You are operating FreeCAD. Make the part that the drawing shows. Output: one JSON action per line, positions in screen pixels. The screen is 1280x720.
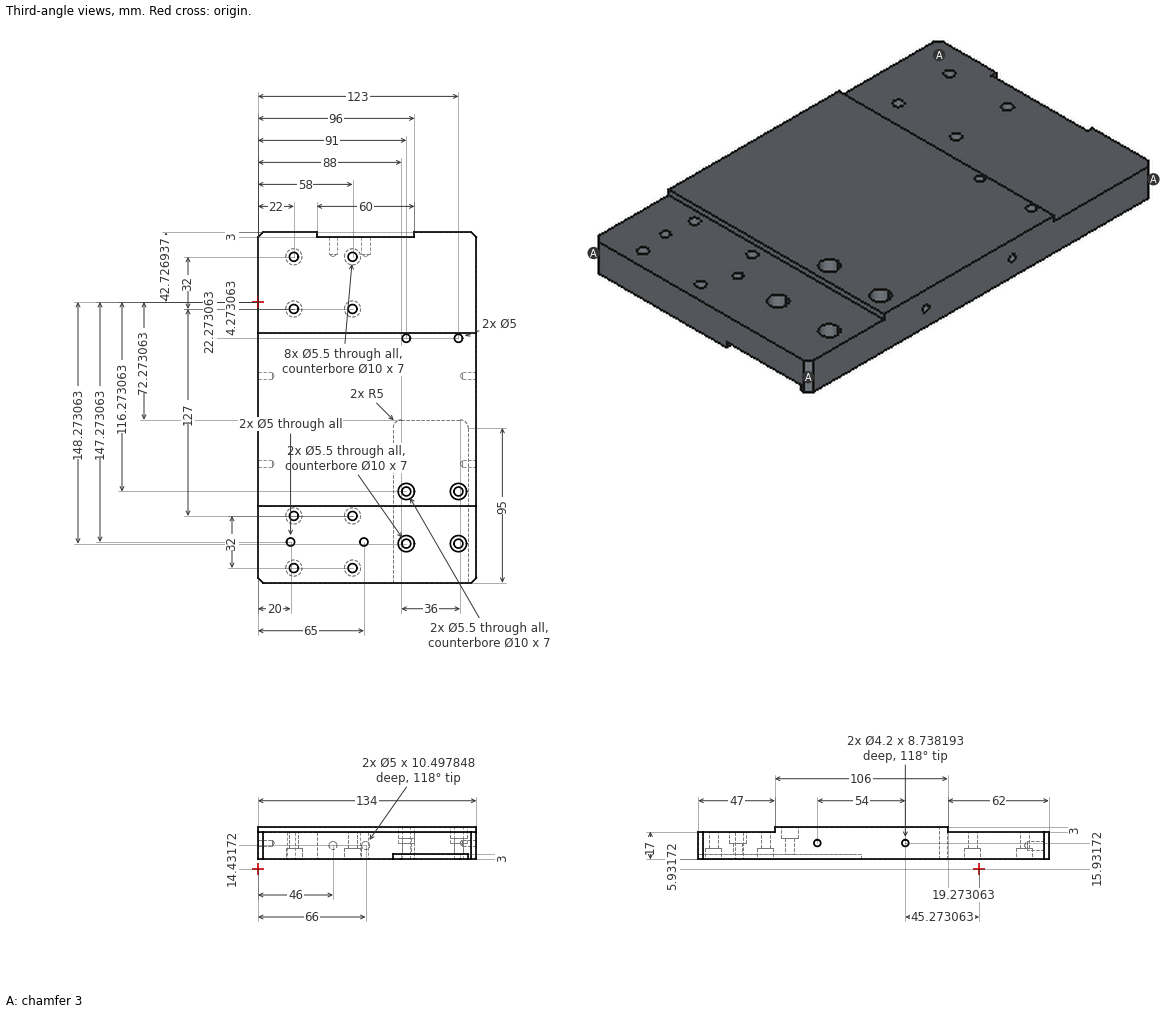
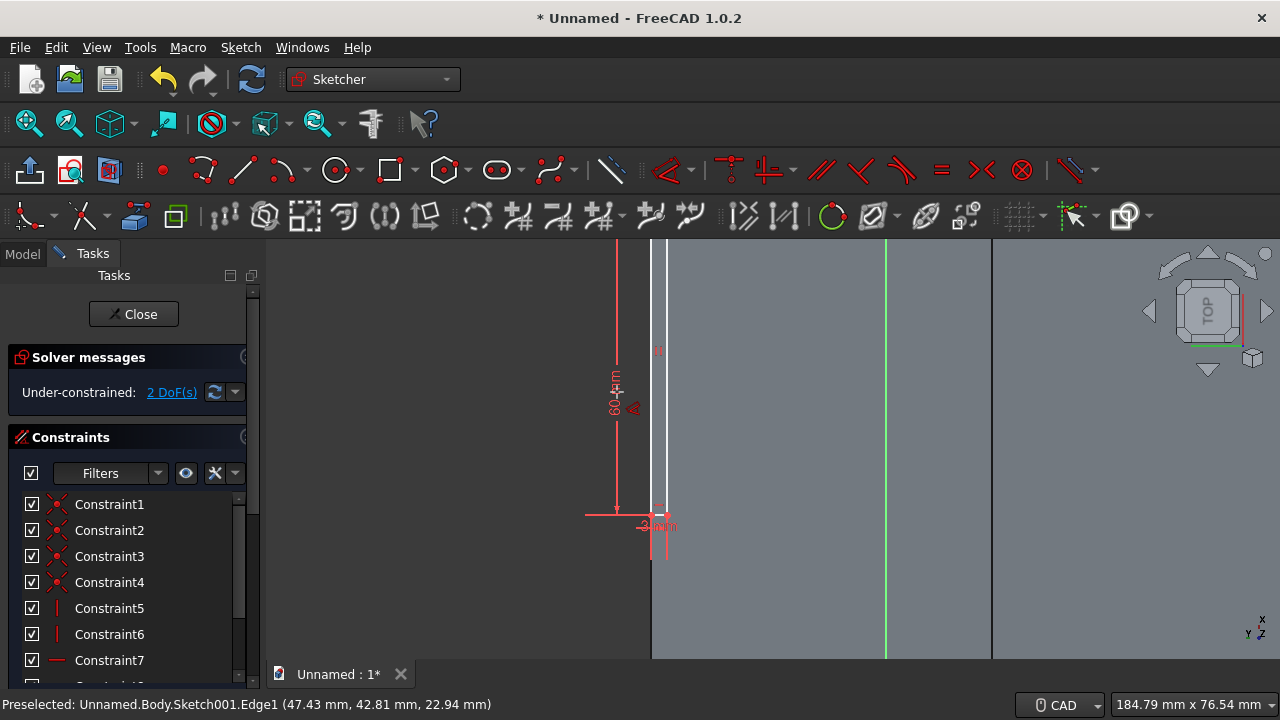
{"action": "scroll", "coordinate": [652, 450], "scroll_direction": "down", "scroll_amount": 4}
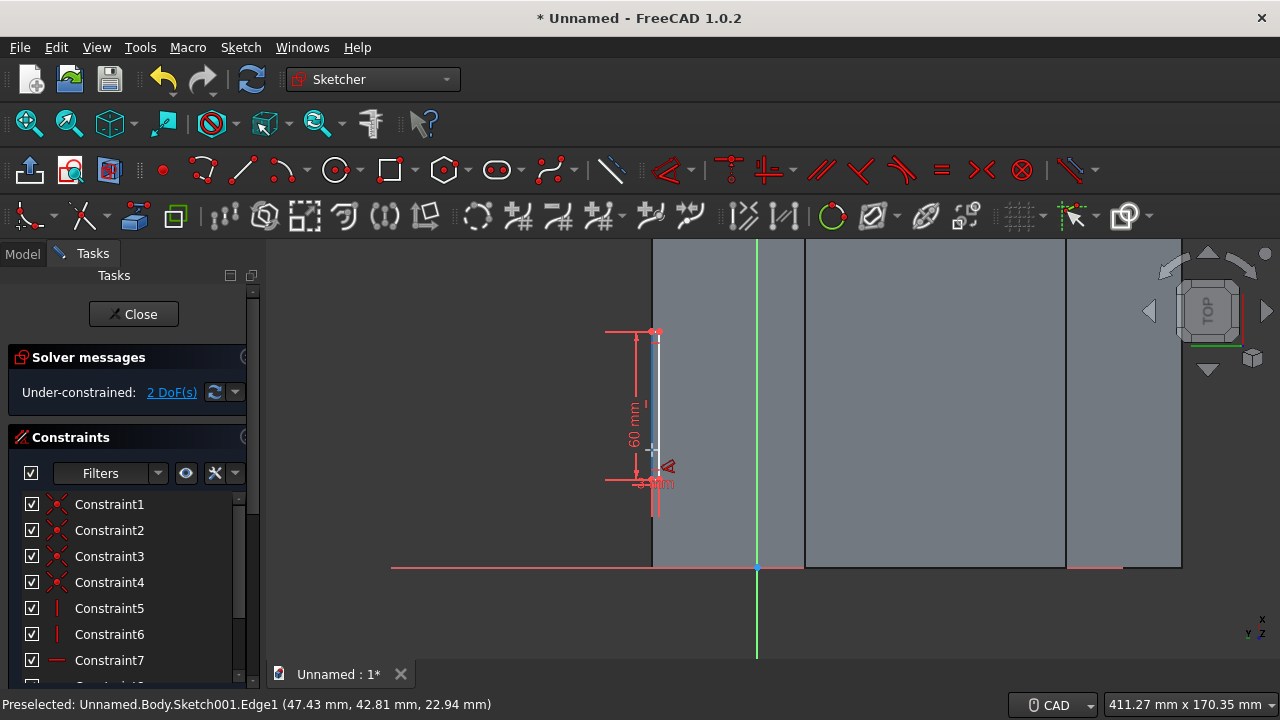
{"action": "scroll", "coordinate": [652, 332], "scroll_direction": "up", "scroll_amount": 3}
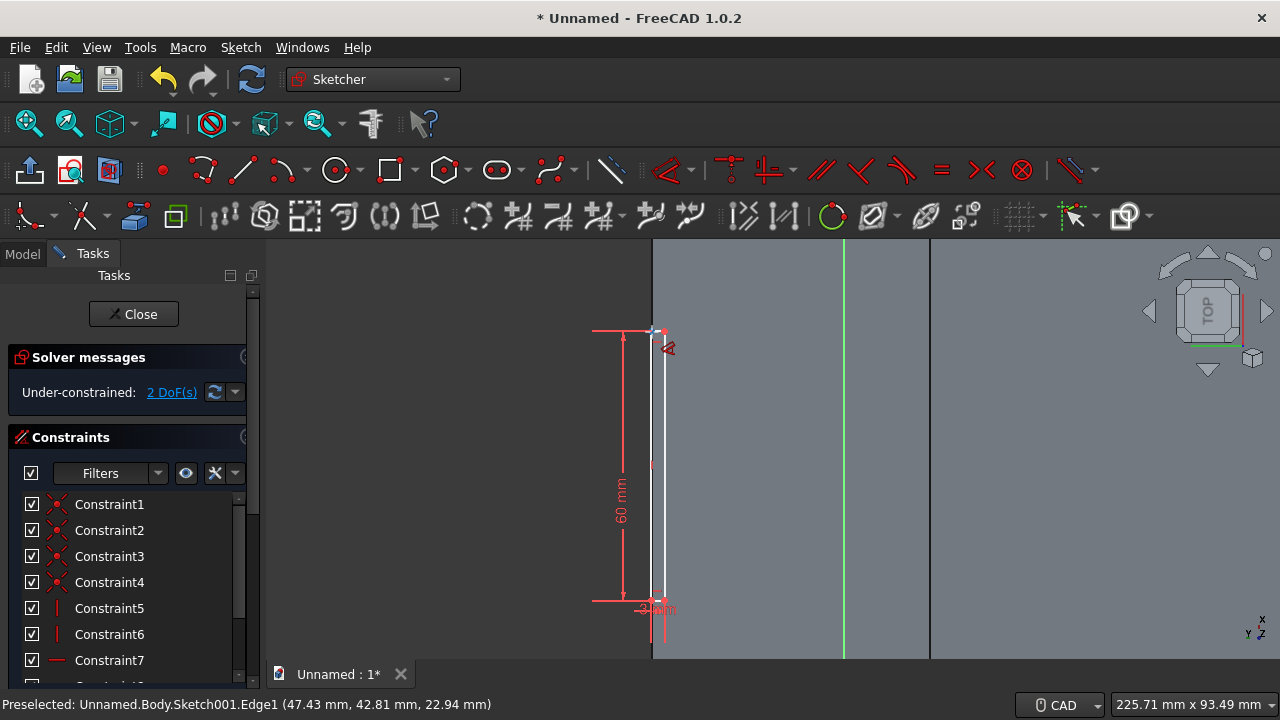
{"action": "left_click", "coordinate": [651, 331]}
{"action": "left_click", "coordinate": [617, 412]}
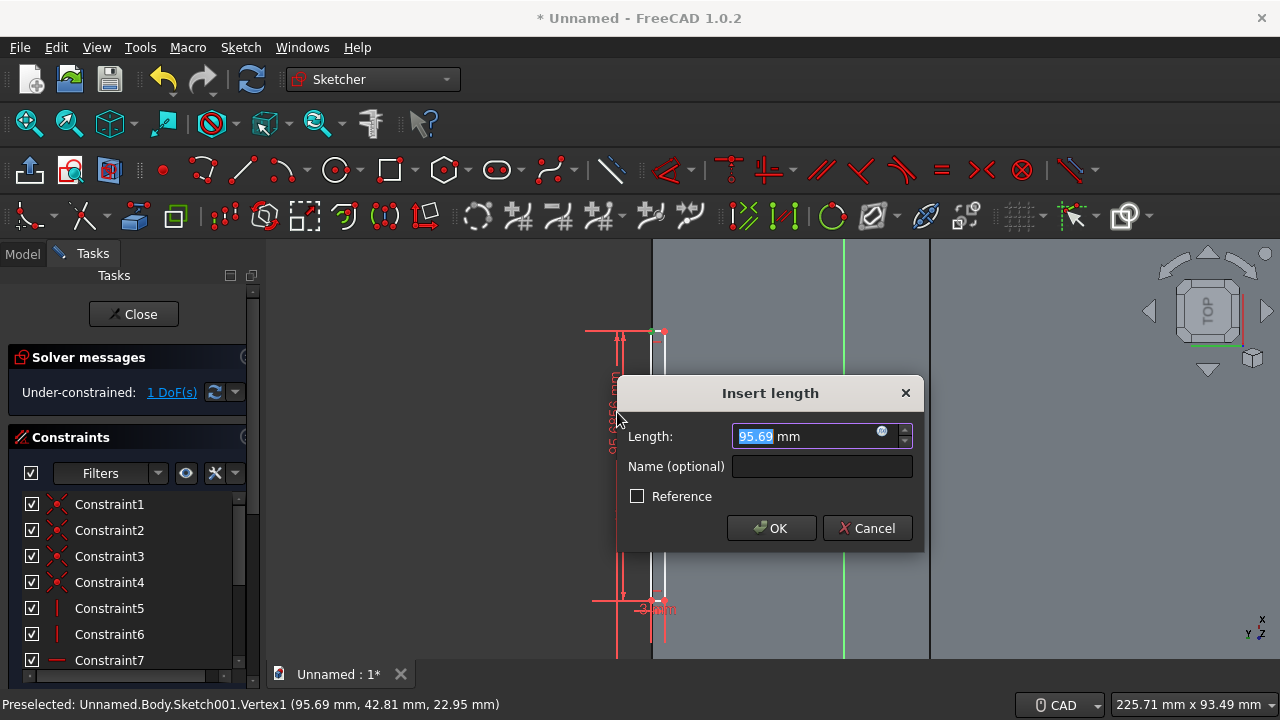
{"action": "type", "text": "96"}
{"action": "key", "text": "Return"}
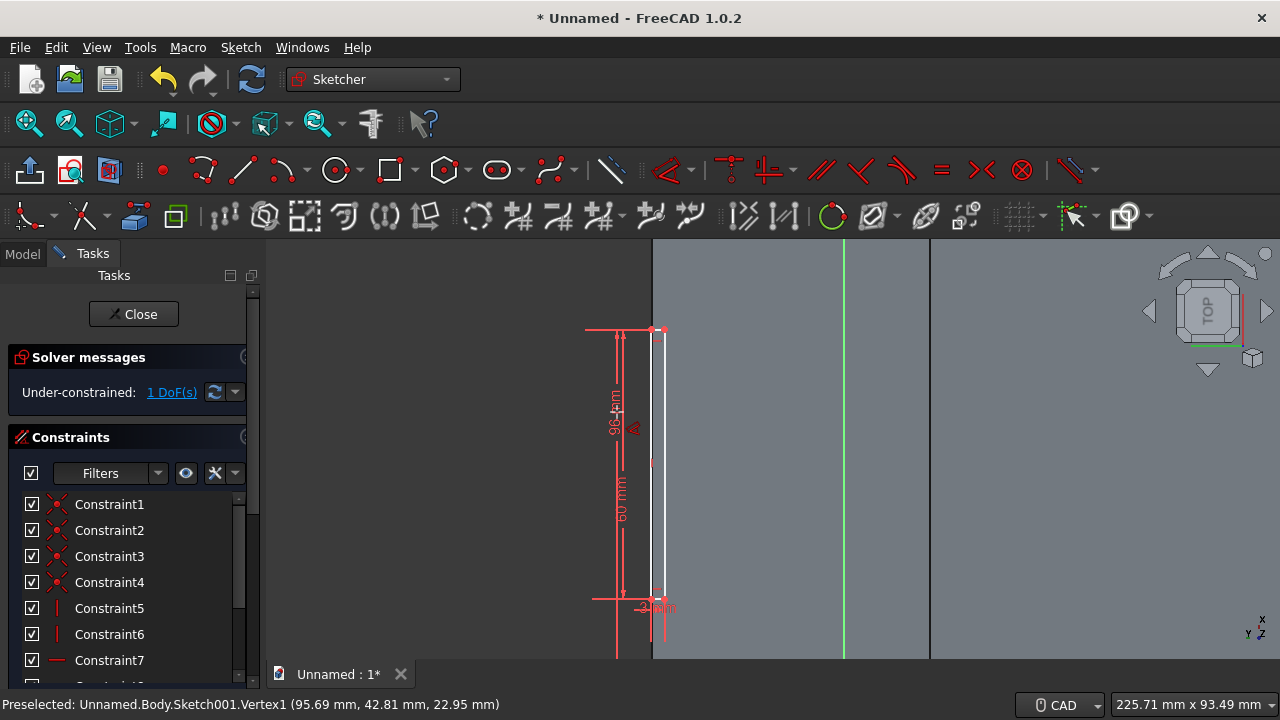
{"action": "left_click", "coordinate": [651, 330]}
{"action": "left_click", "coordinate": [747, 296]}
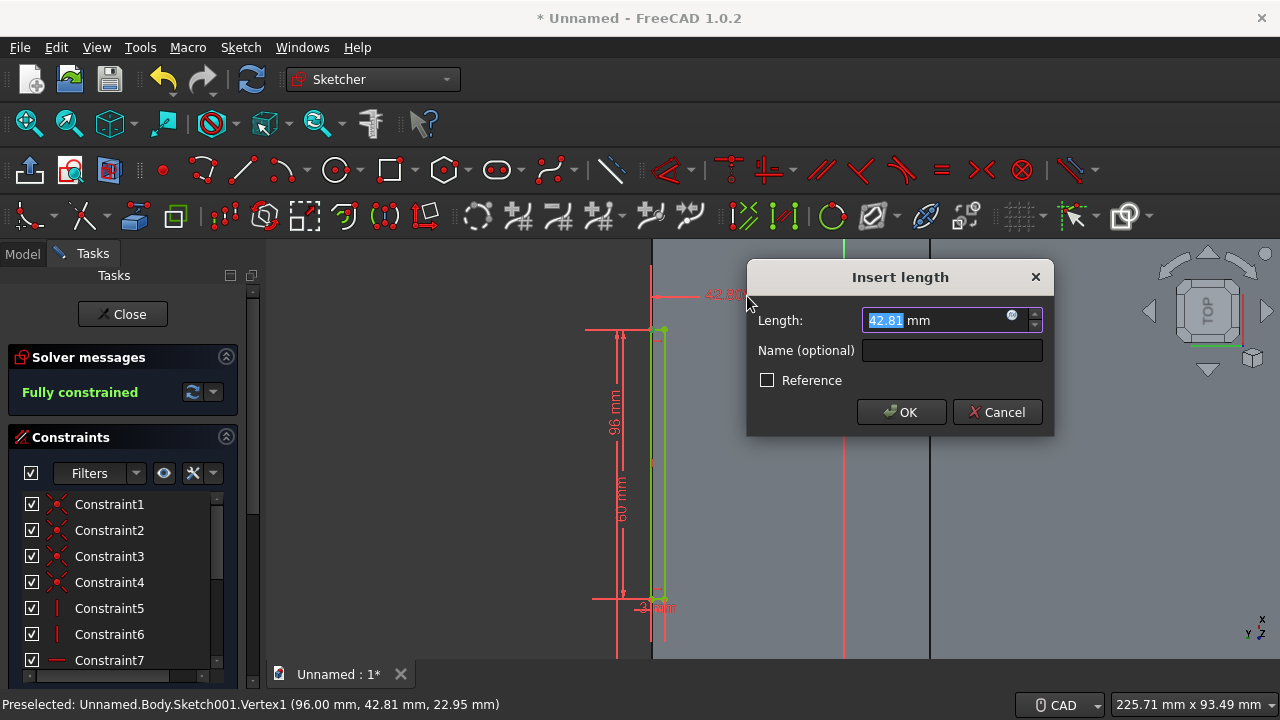
{"action": "type", "text": "42.726937"}
{"action": "key", "text": "Return"}
{"action": "key", "text": "Escape"}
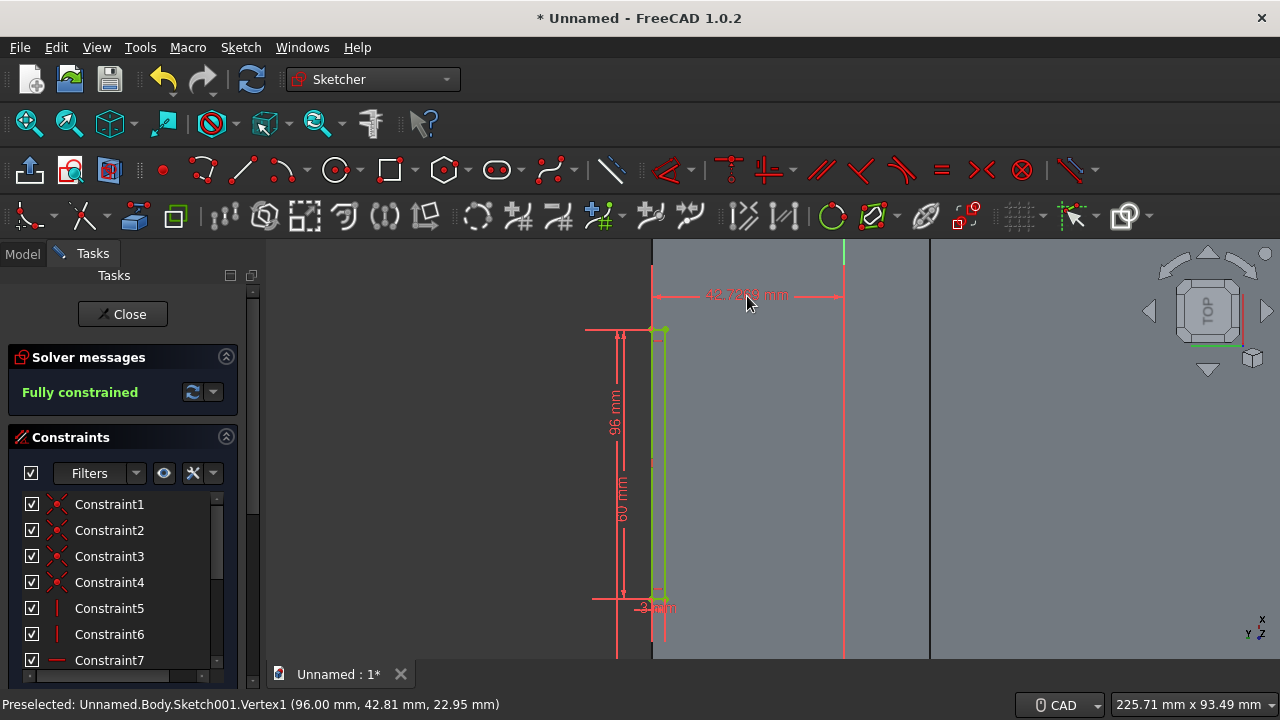
{"action": "left_click", "coordinate": [123, 314]}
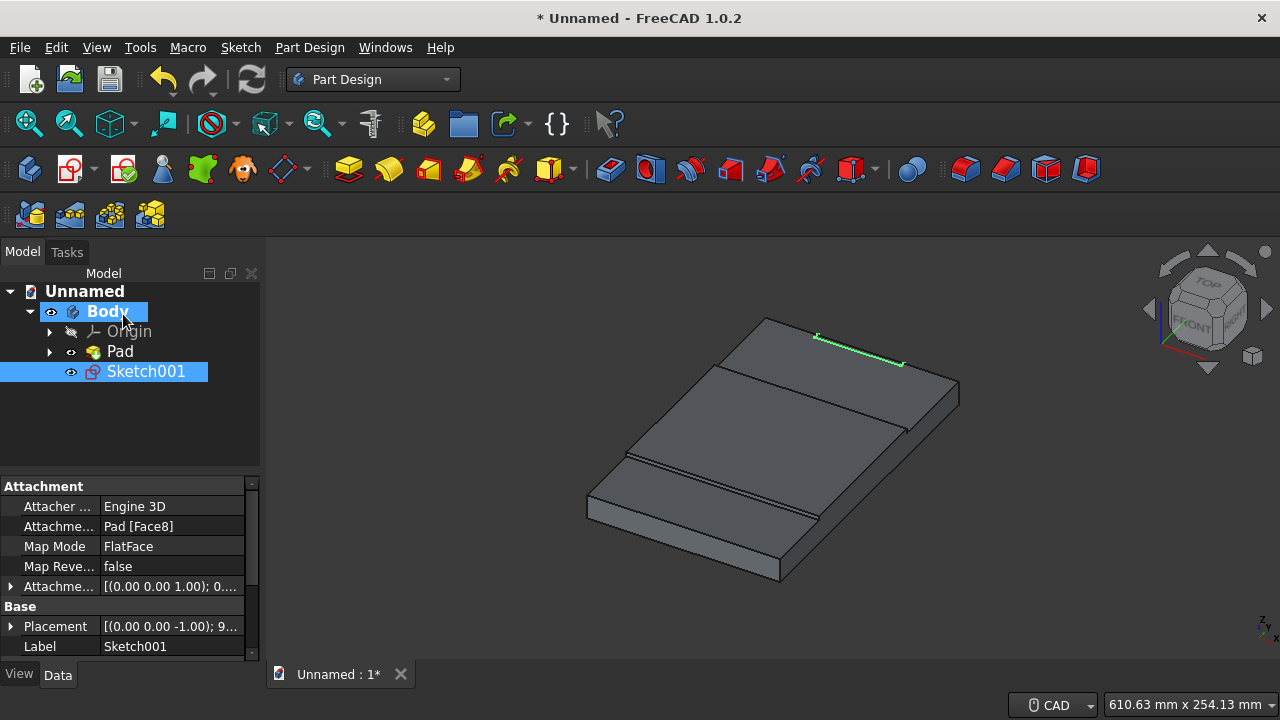
{"action": "left_click", "coordinate": [612, 170]}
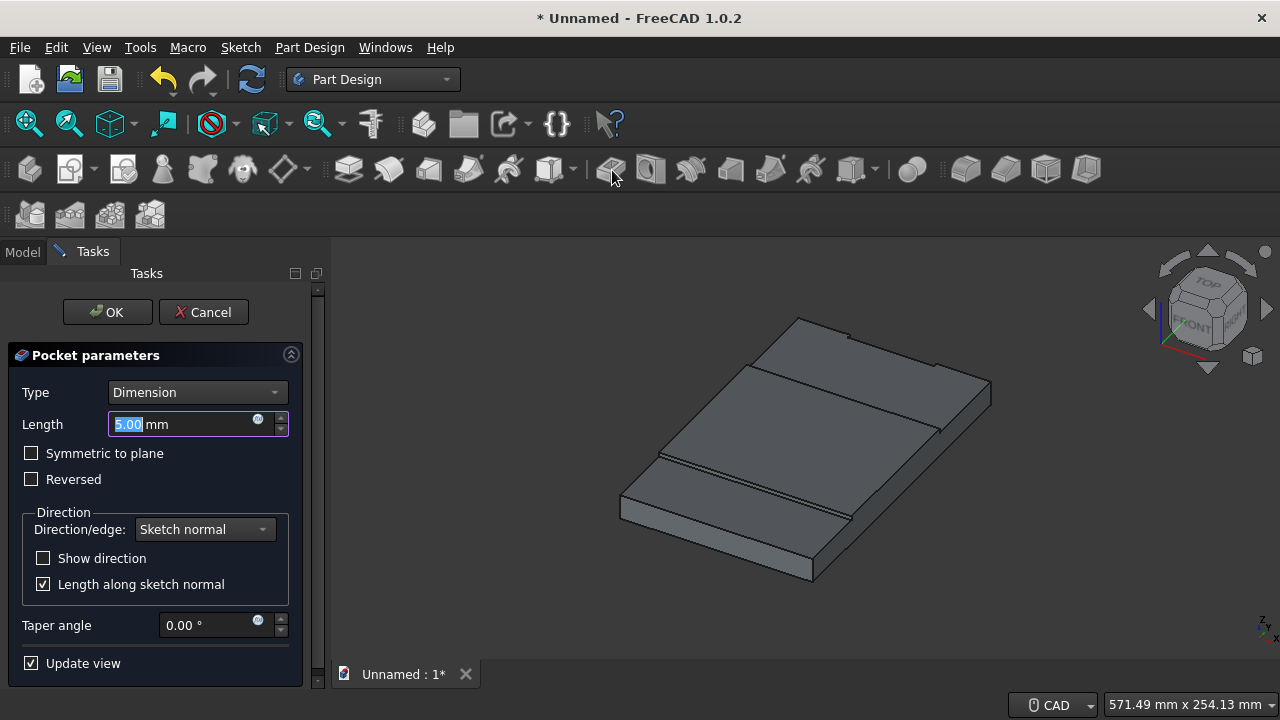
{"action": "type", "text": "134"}
{"action": "key", "text": "Tab"}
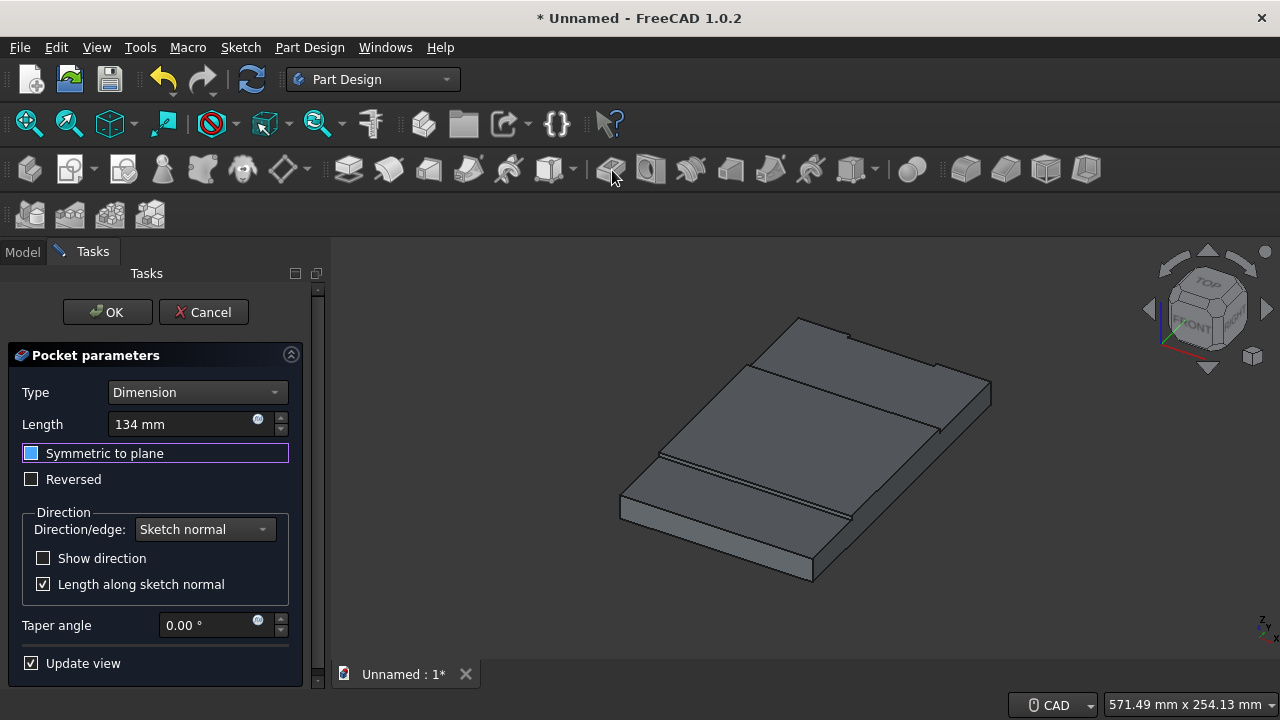
{"action": "left_click", "coordinate": [108, 312]}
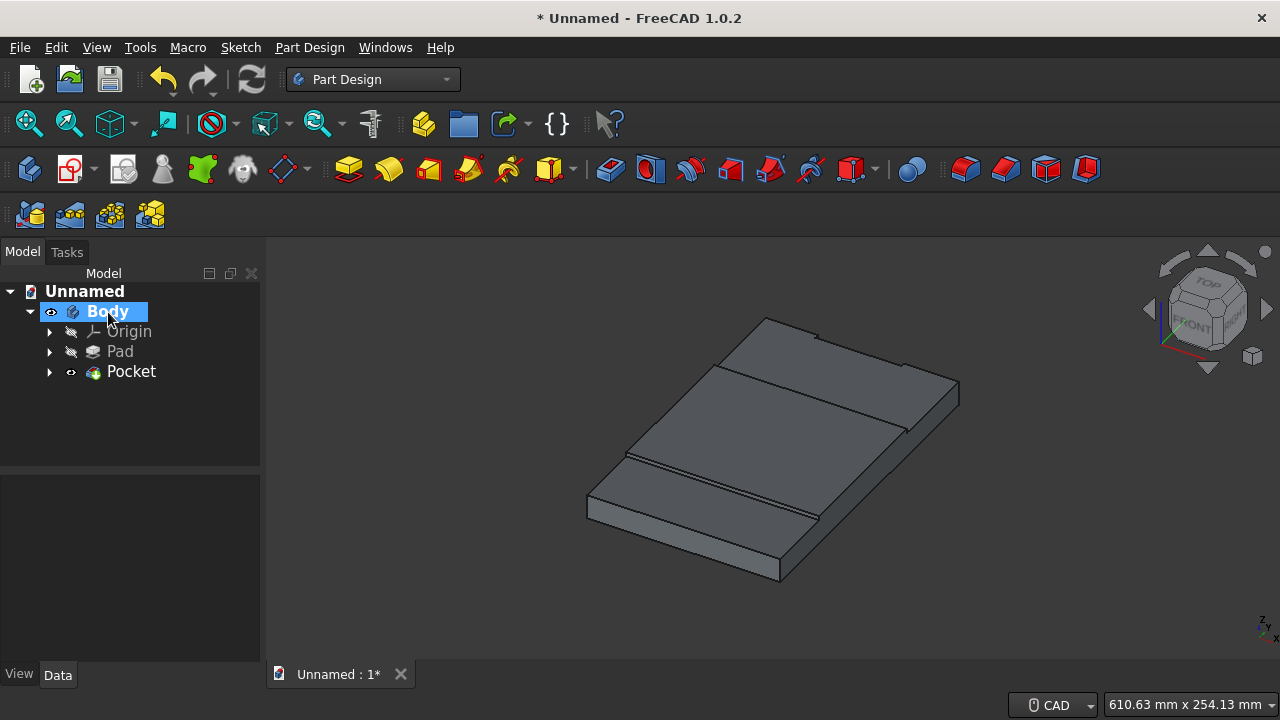
{"action": "left_click", "coordinate": [780, 570]}